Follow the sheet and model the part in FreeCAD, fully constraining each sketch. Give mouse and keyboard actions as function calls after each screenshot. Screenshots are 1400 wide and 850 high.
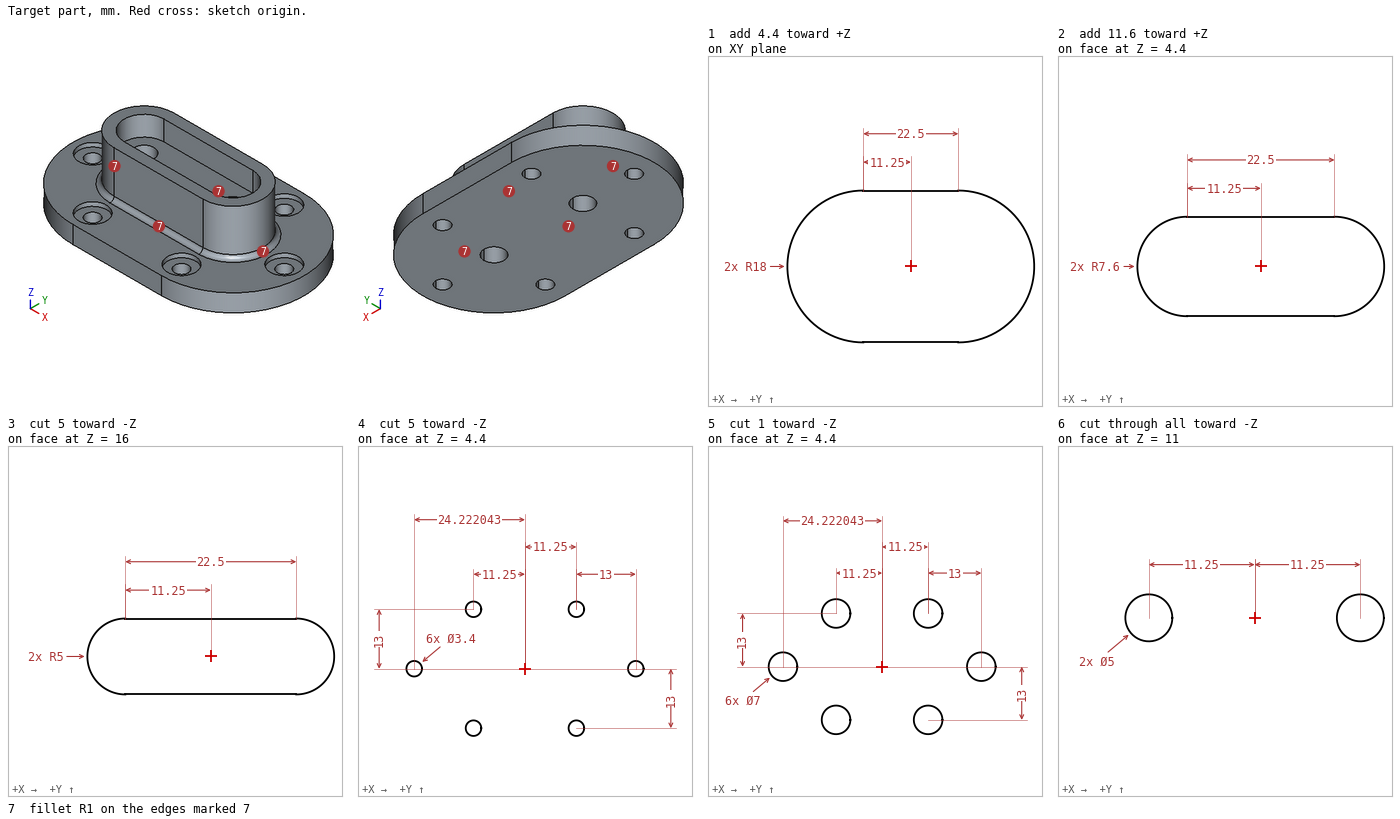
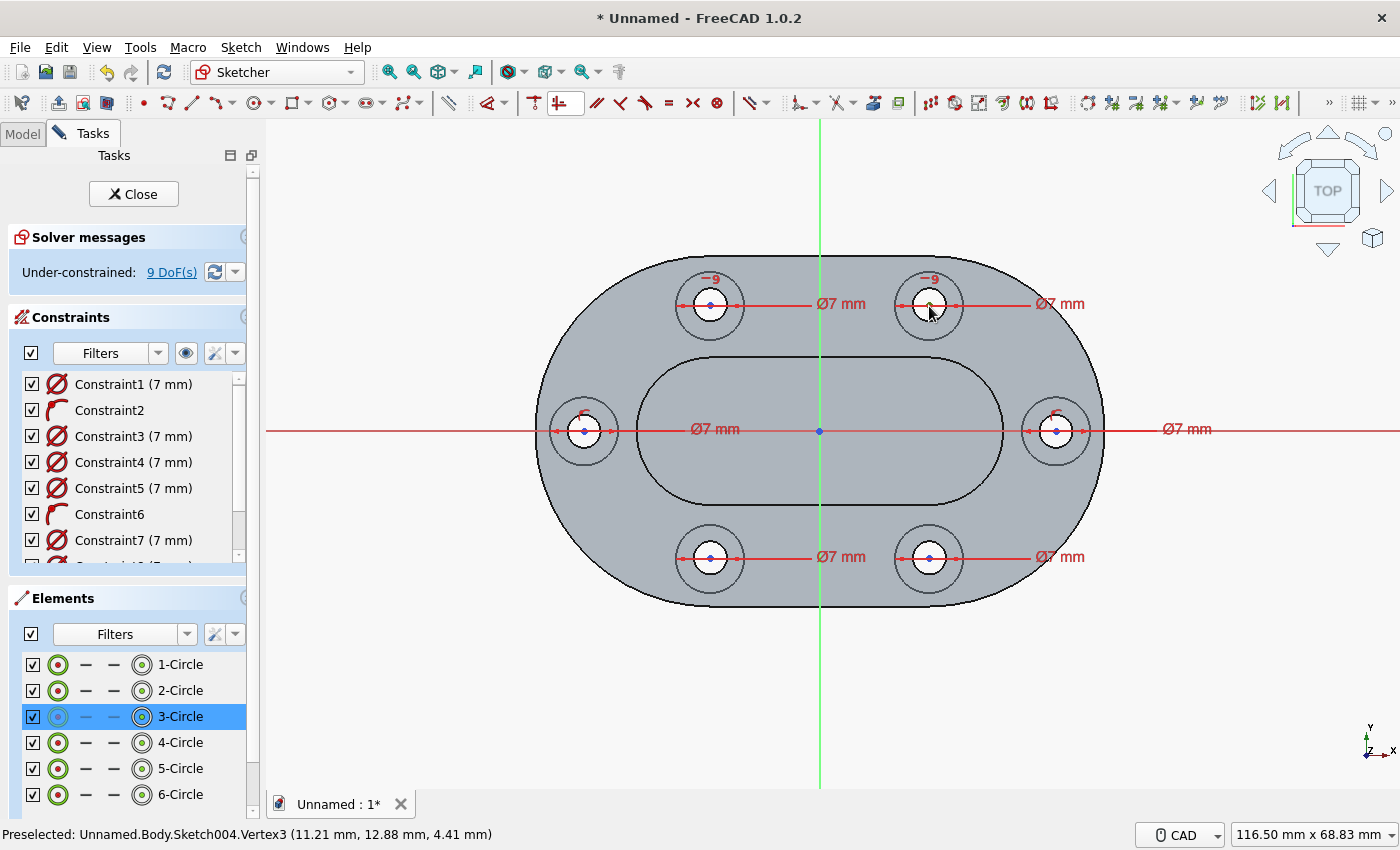
click(929, 559)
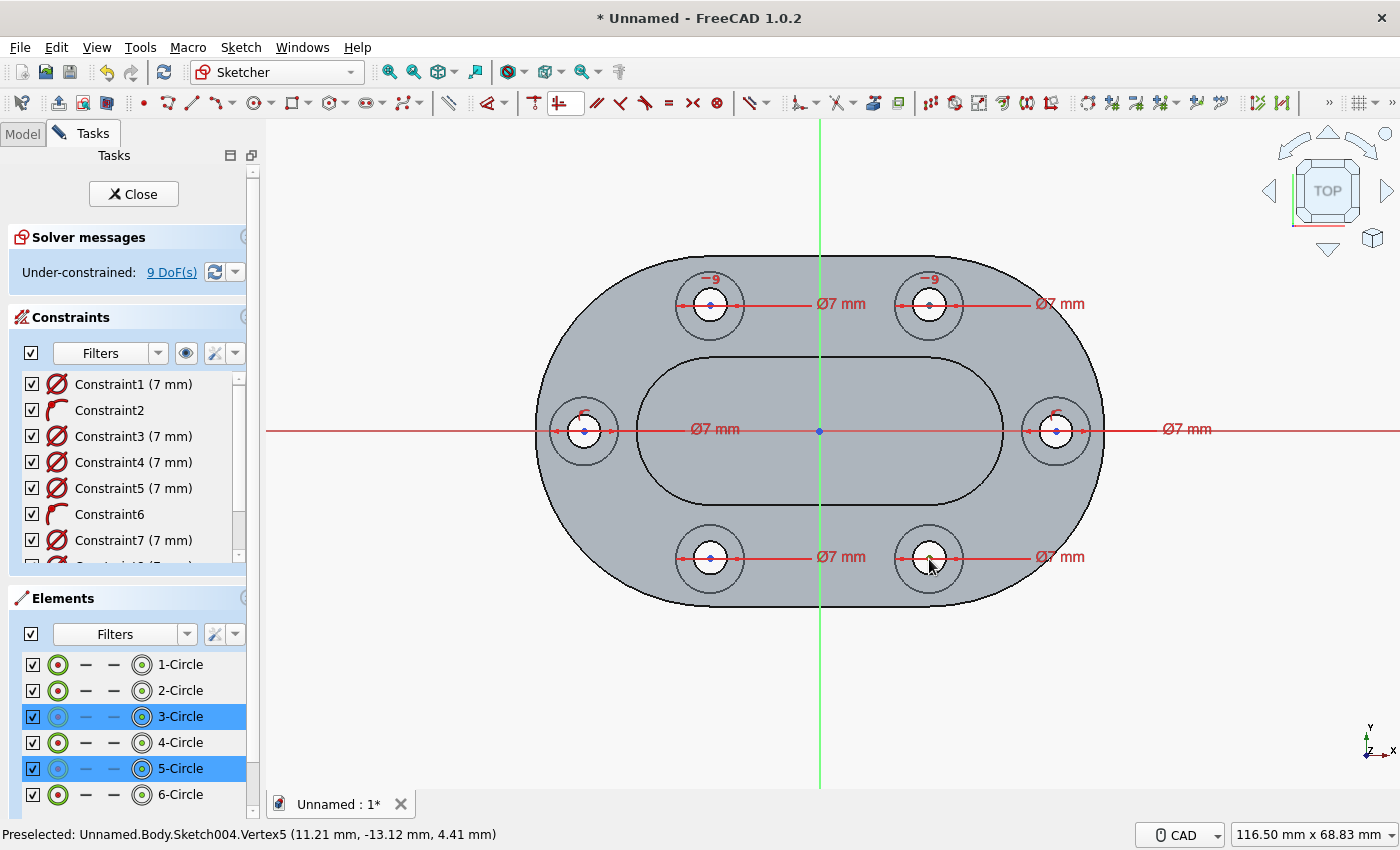
click(578, 104)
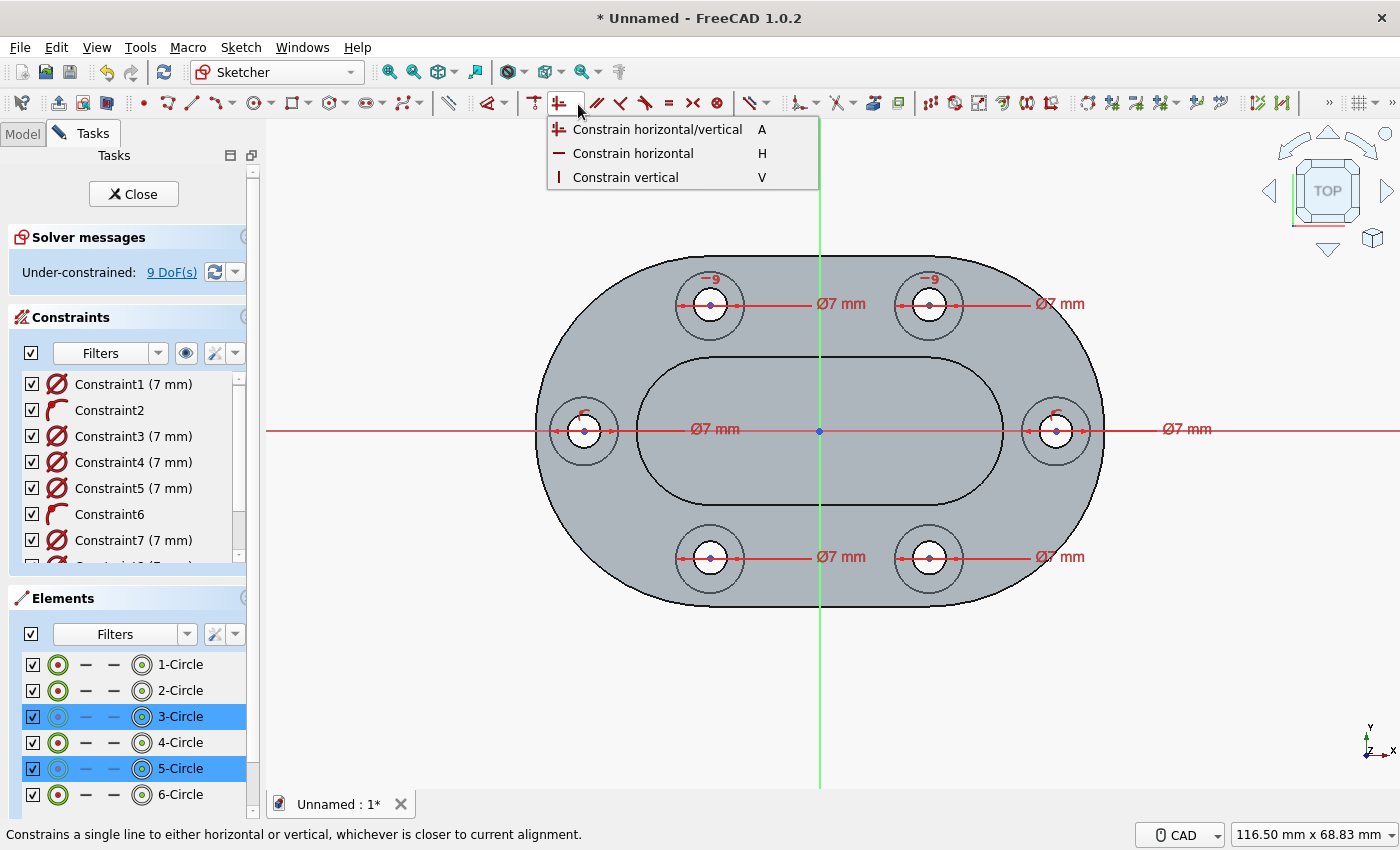
click(683, 177)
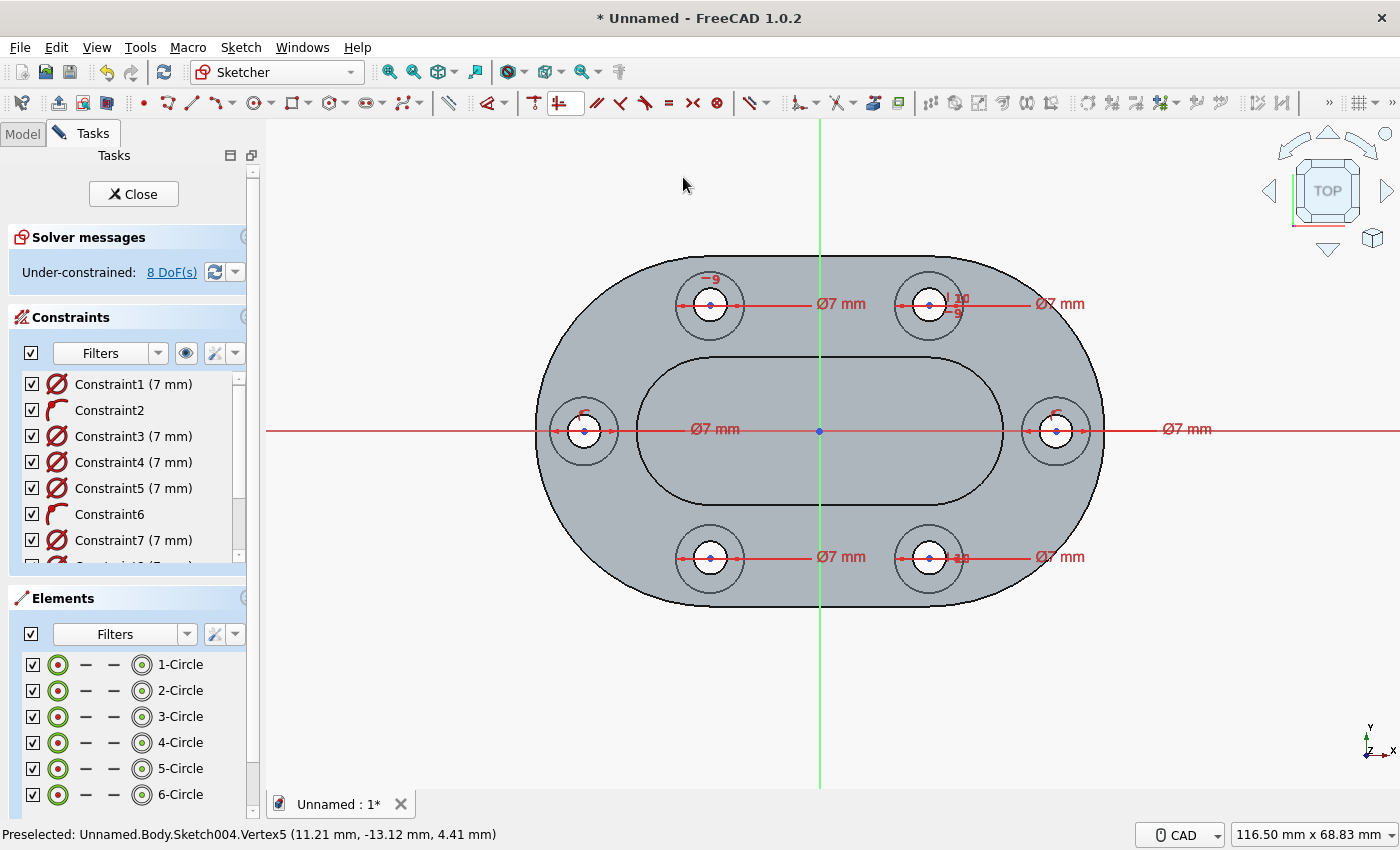
click(710, 306)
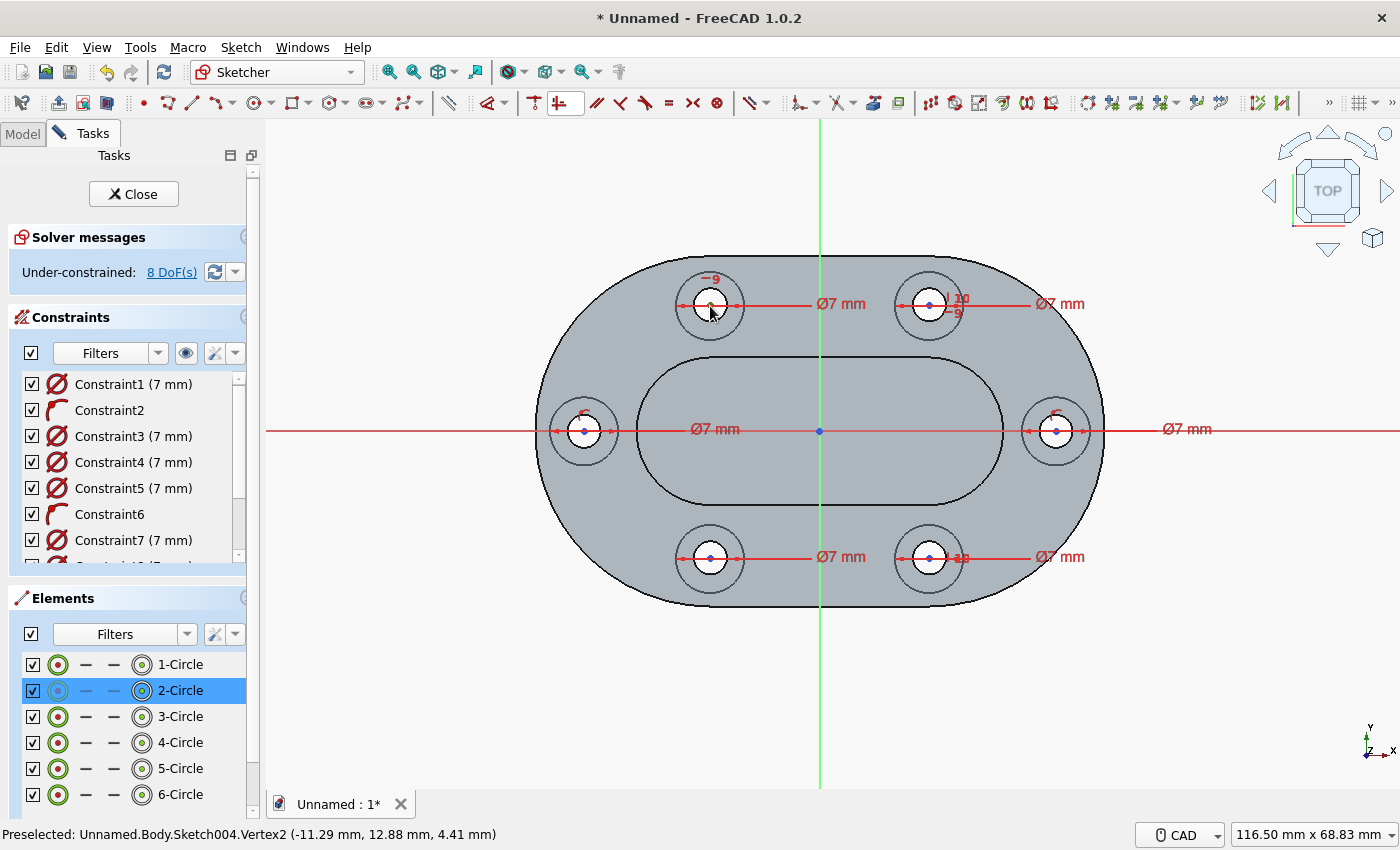
click(710, 559)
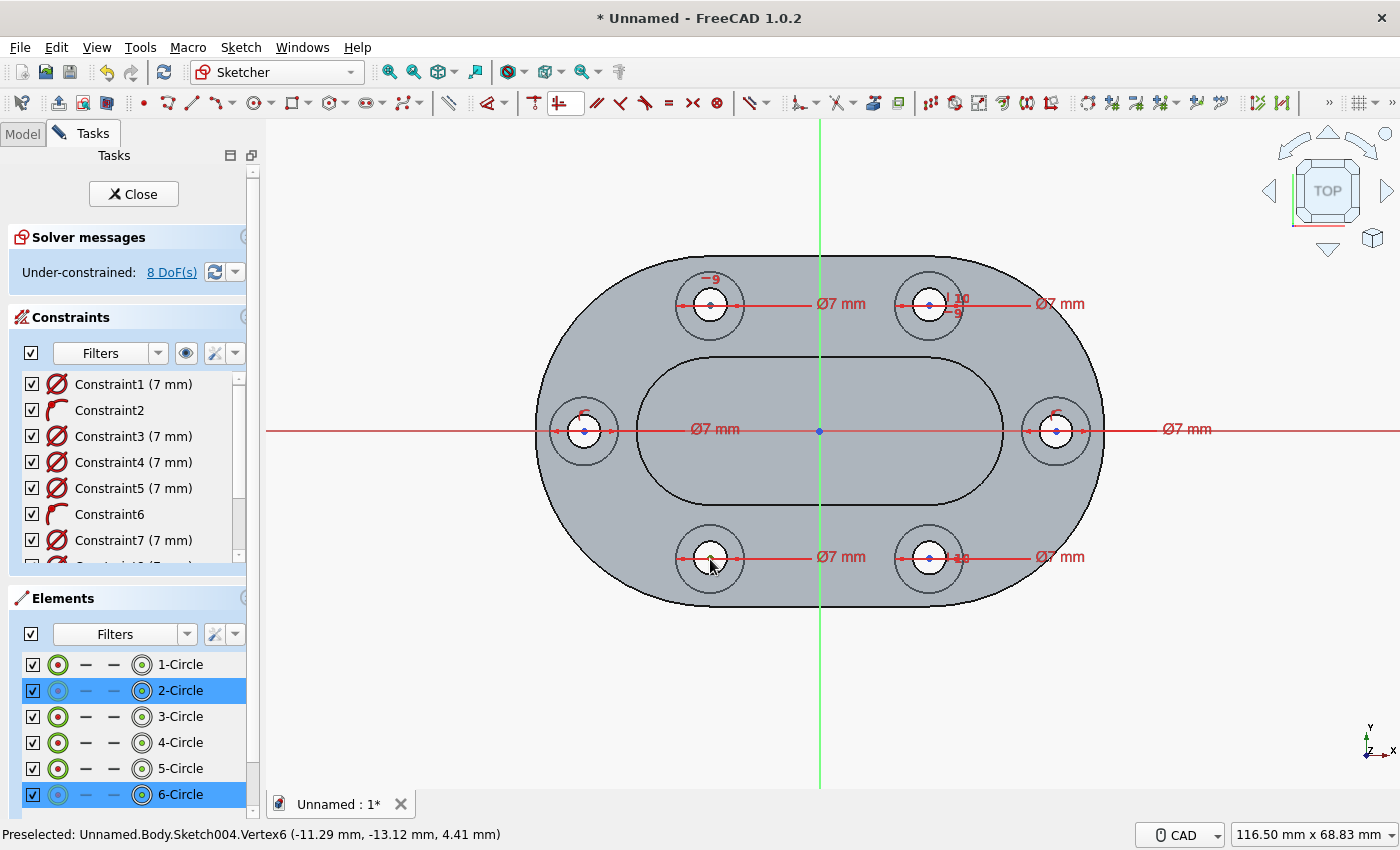
key(v)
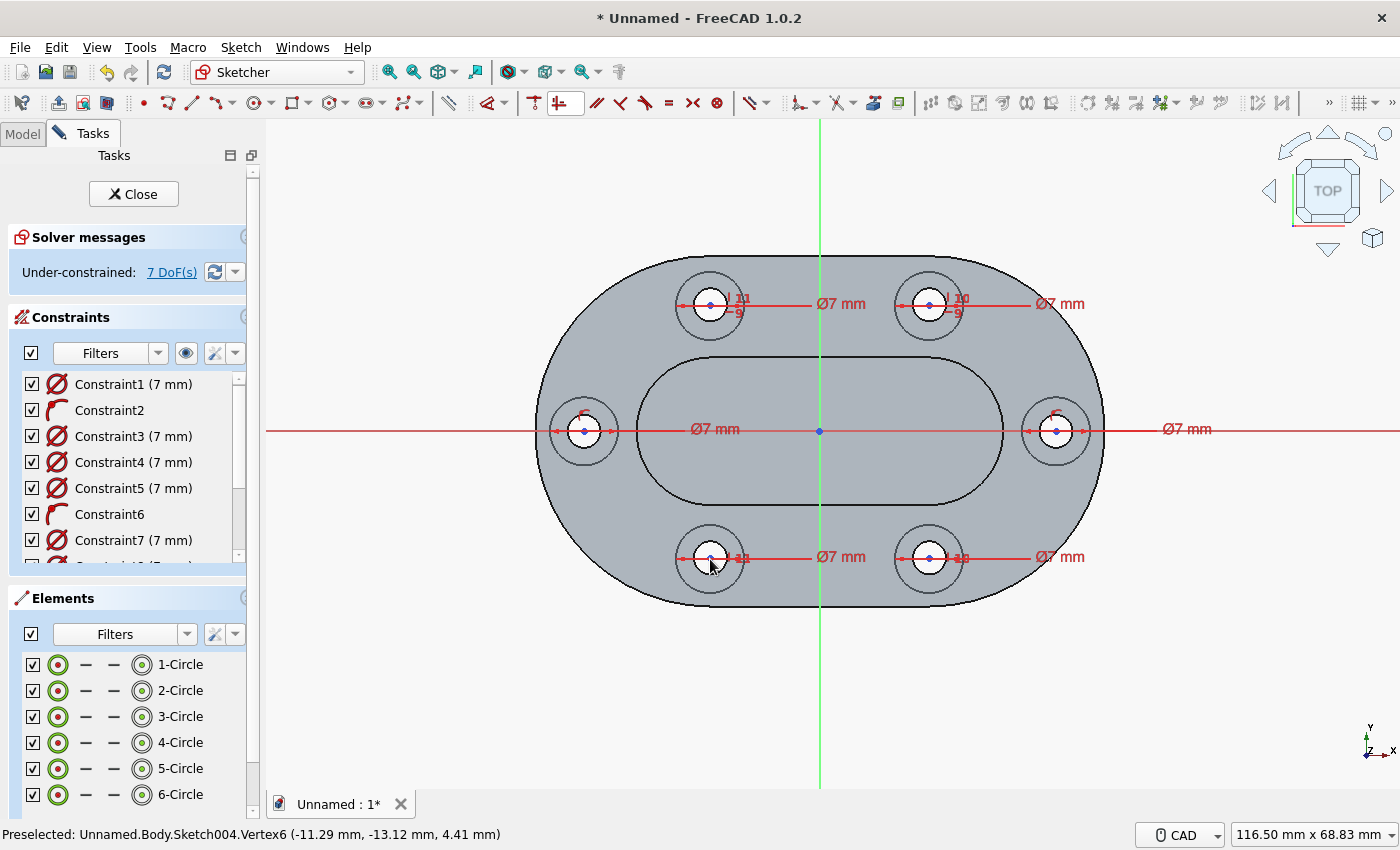
click(929, 559)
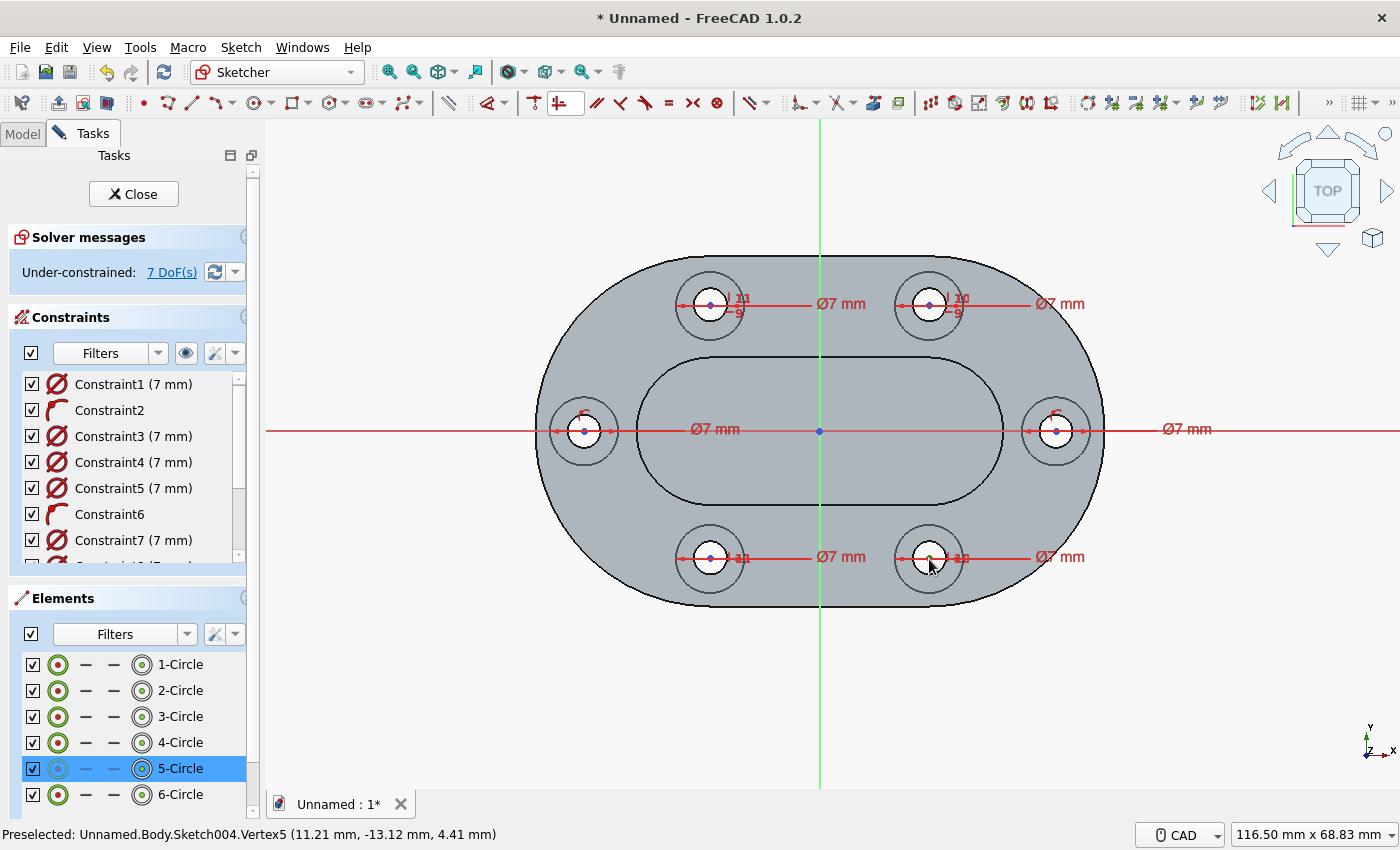
click(710, 559)